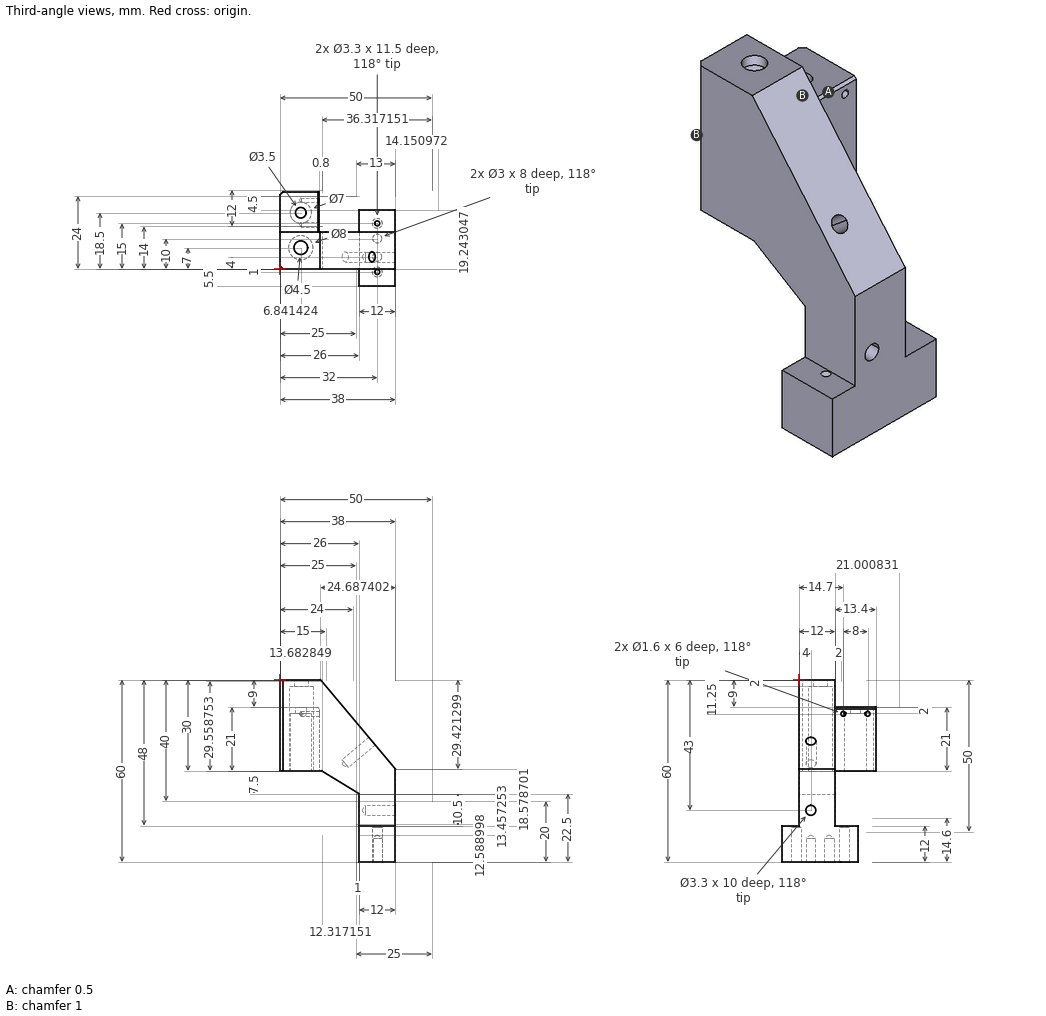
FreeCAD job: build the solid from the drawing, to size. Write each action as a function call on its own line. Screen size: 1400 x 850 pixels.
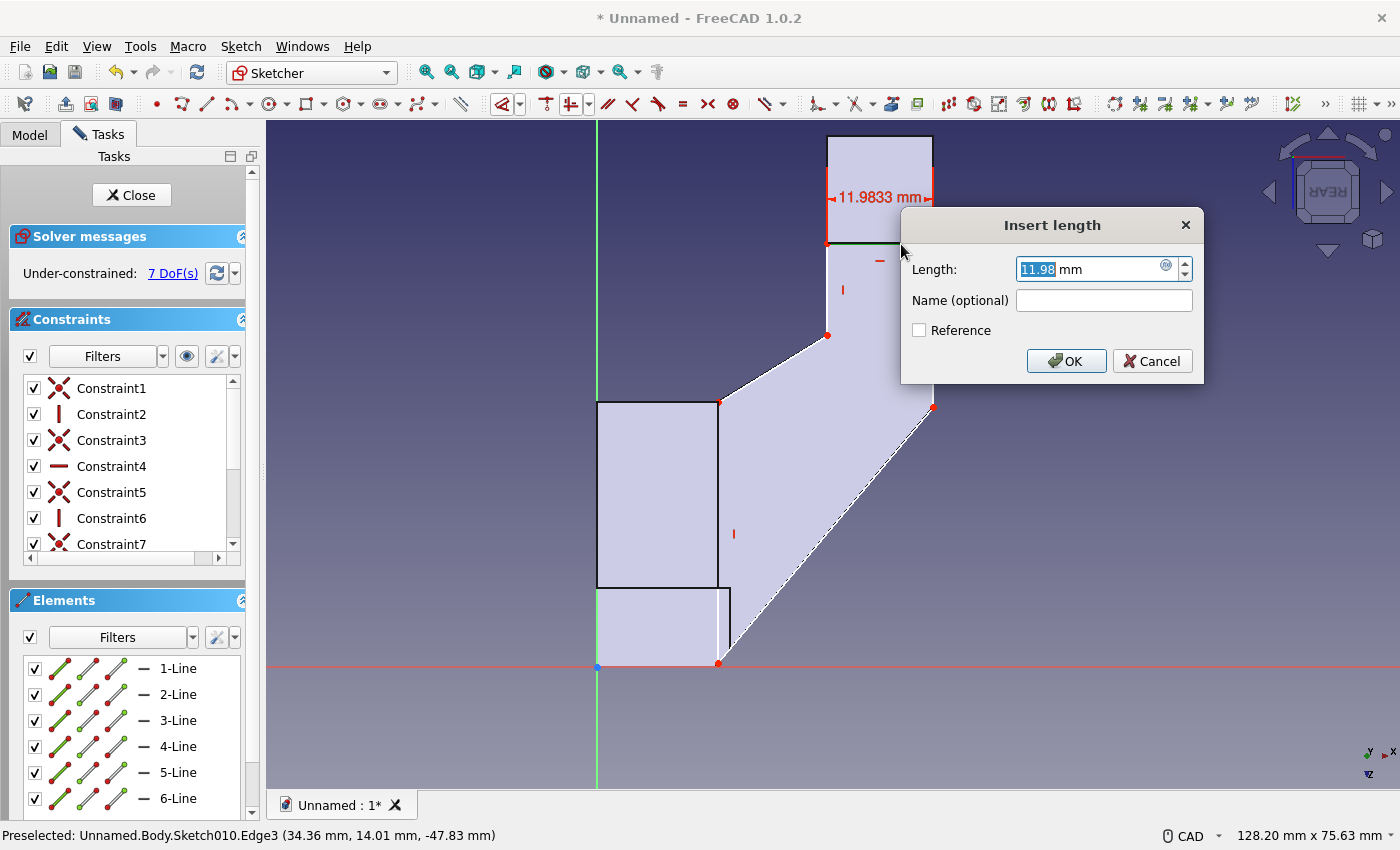
text(12)
key(Return)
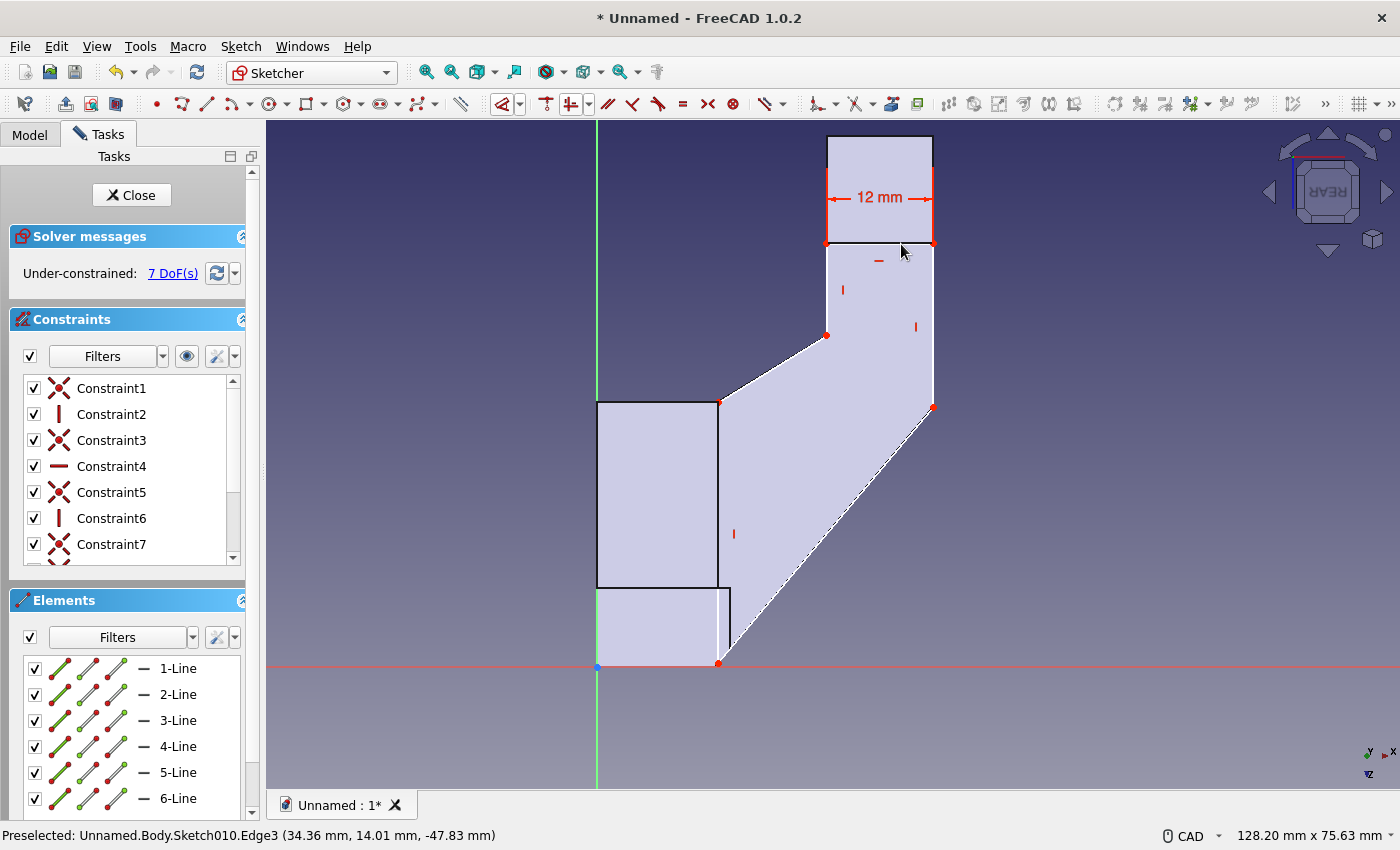
click(933, 408)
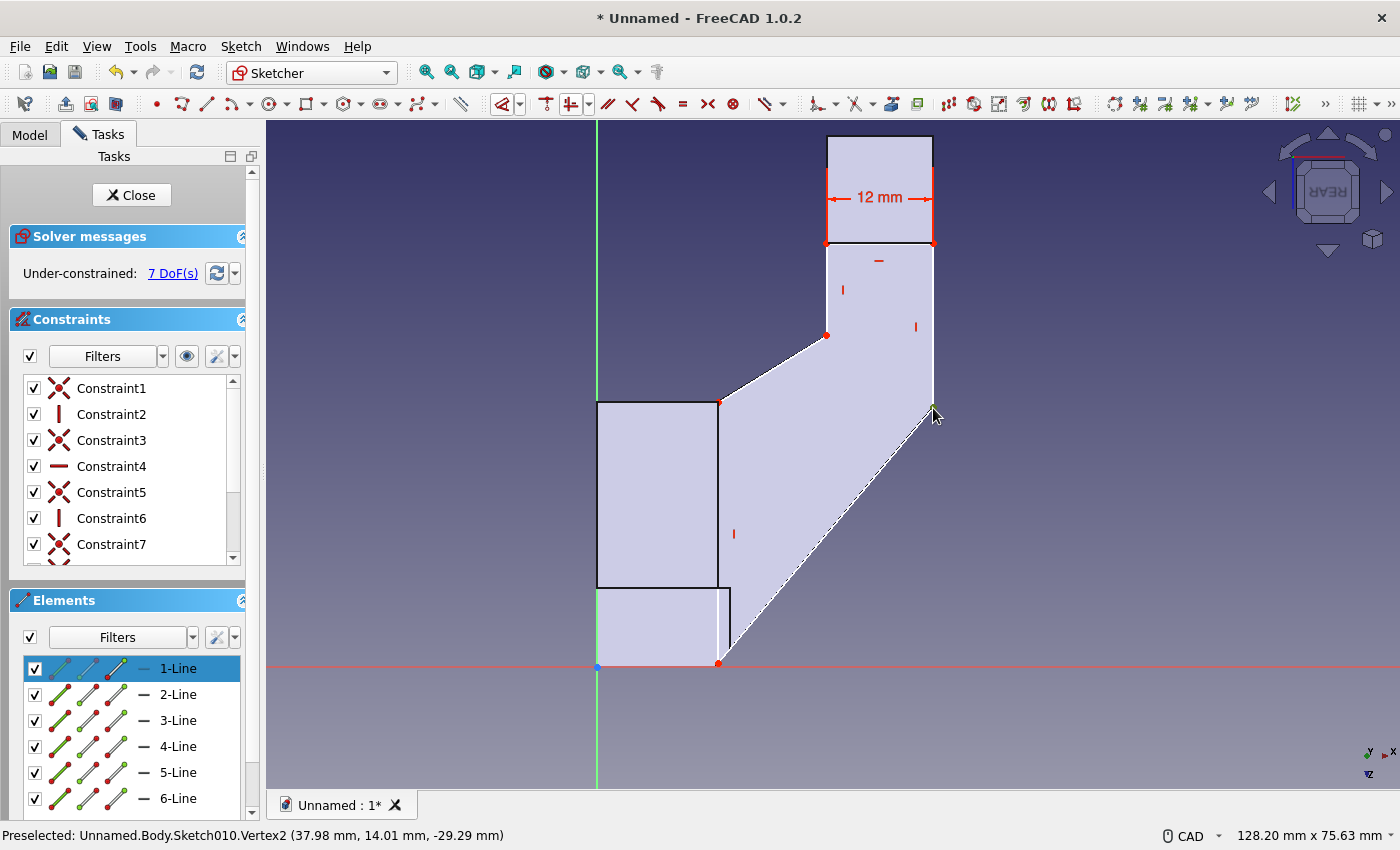
click(520, 104)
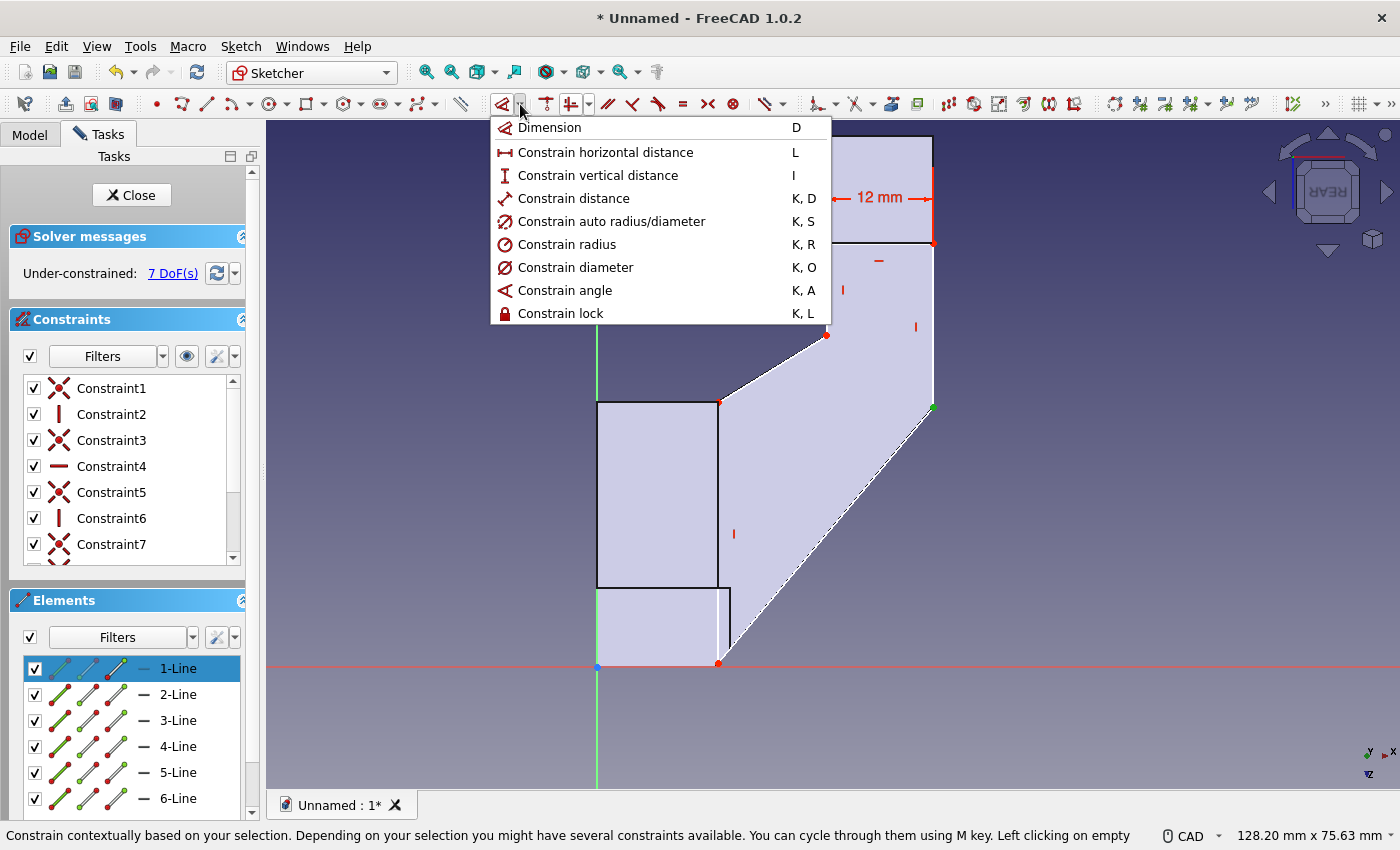
click(661, 152)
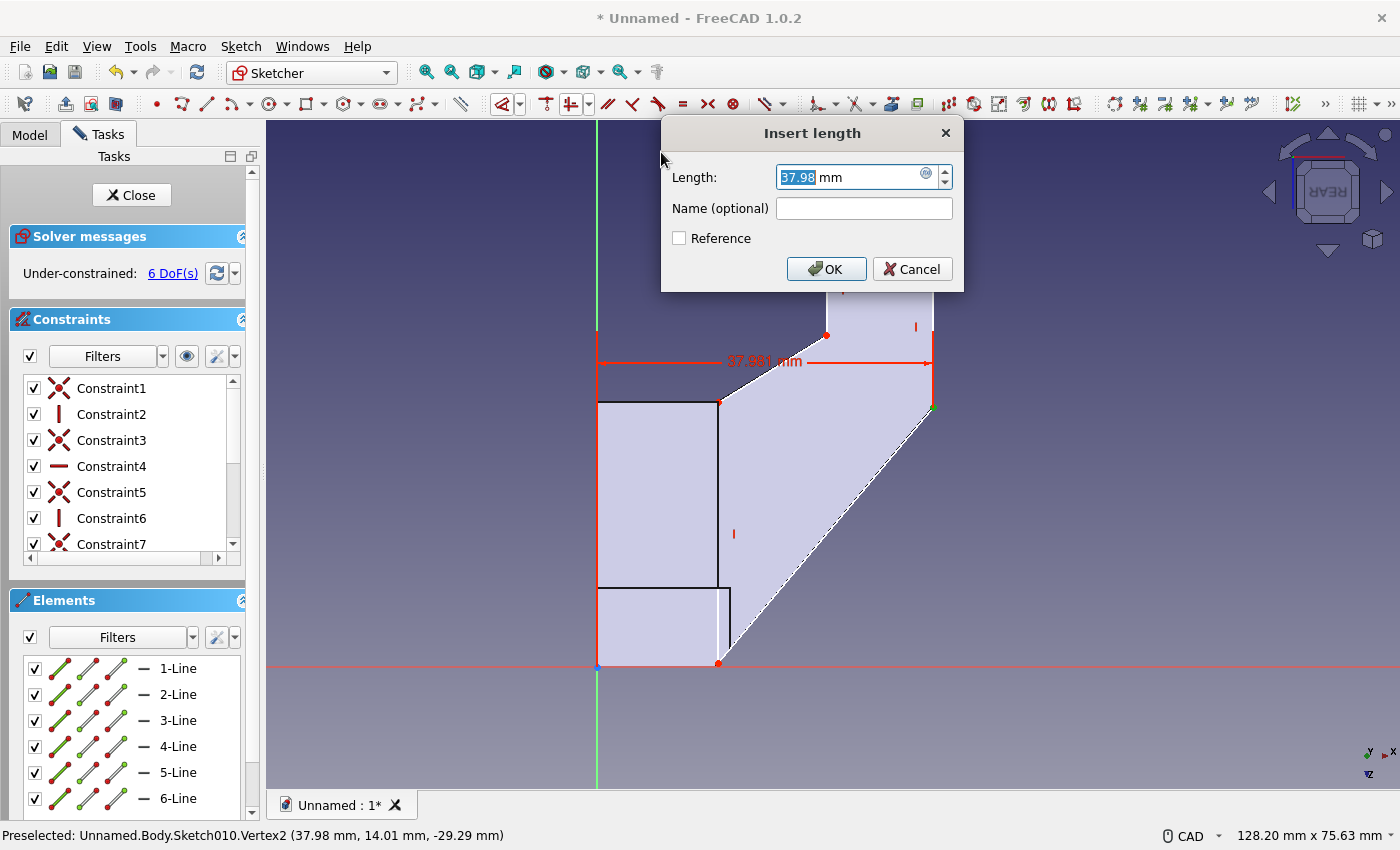
text(38)
key(Return)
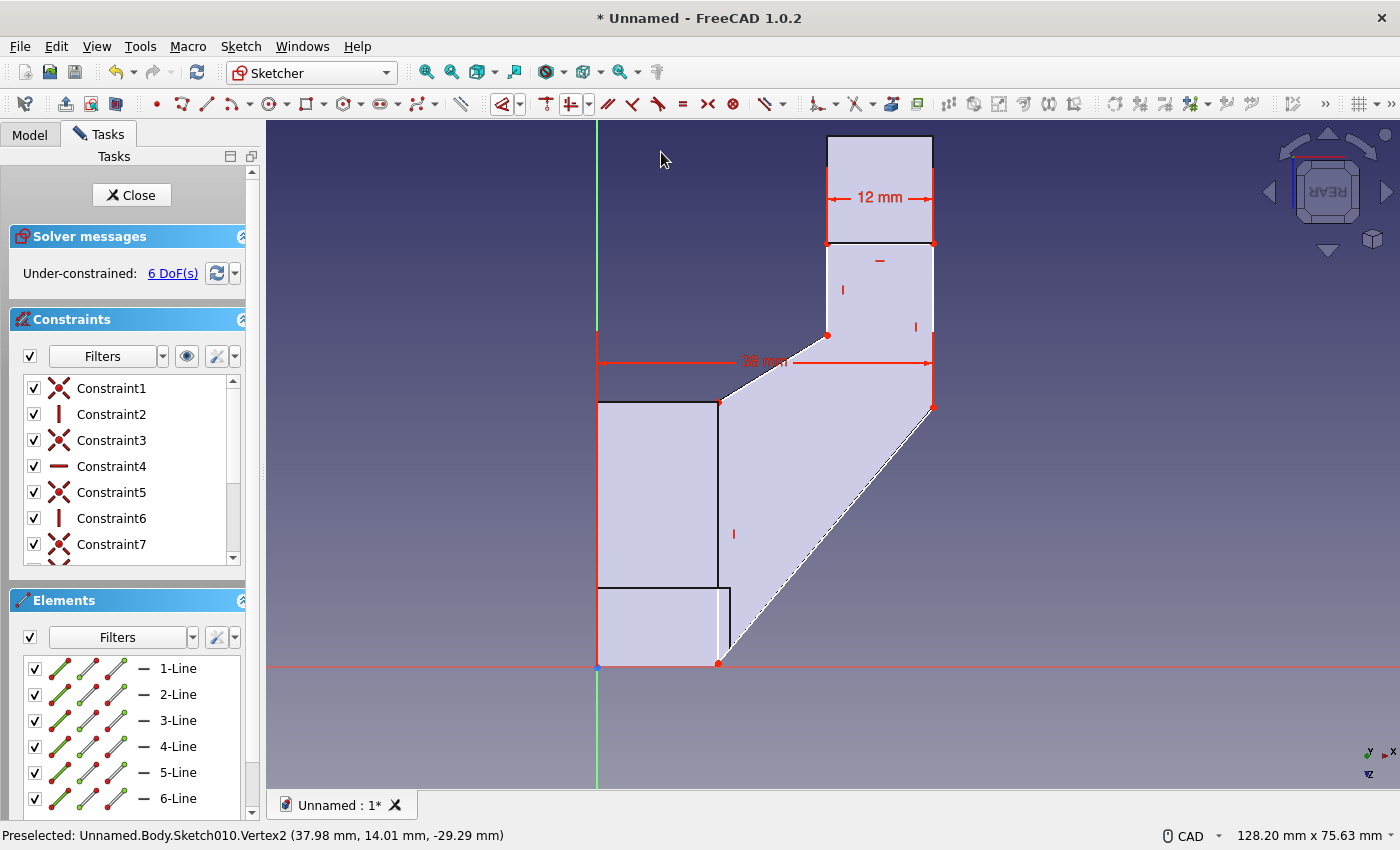
click(933, 244)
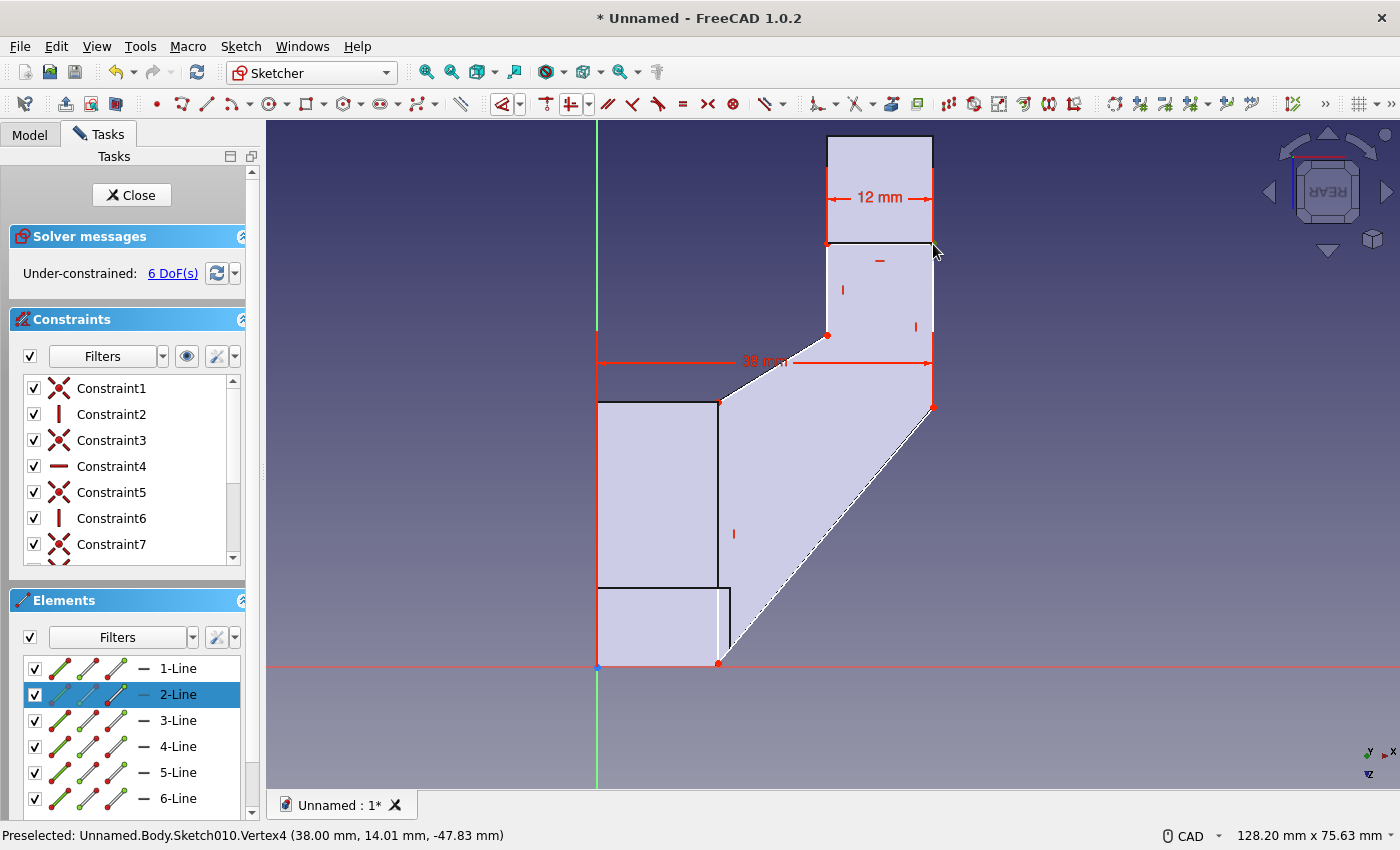
key(i)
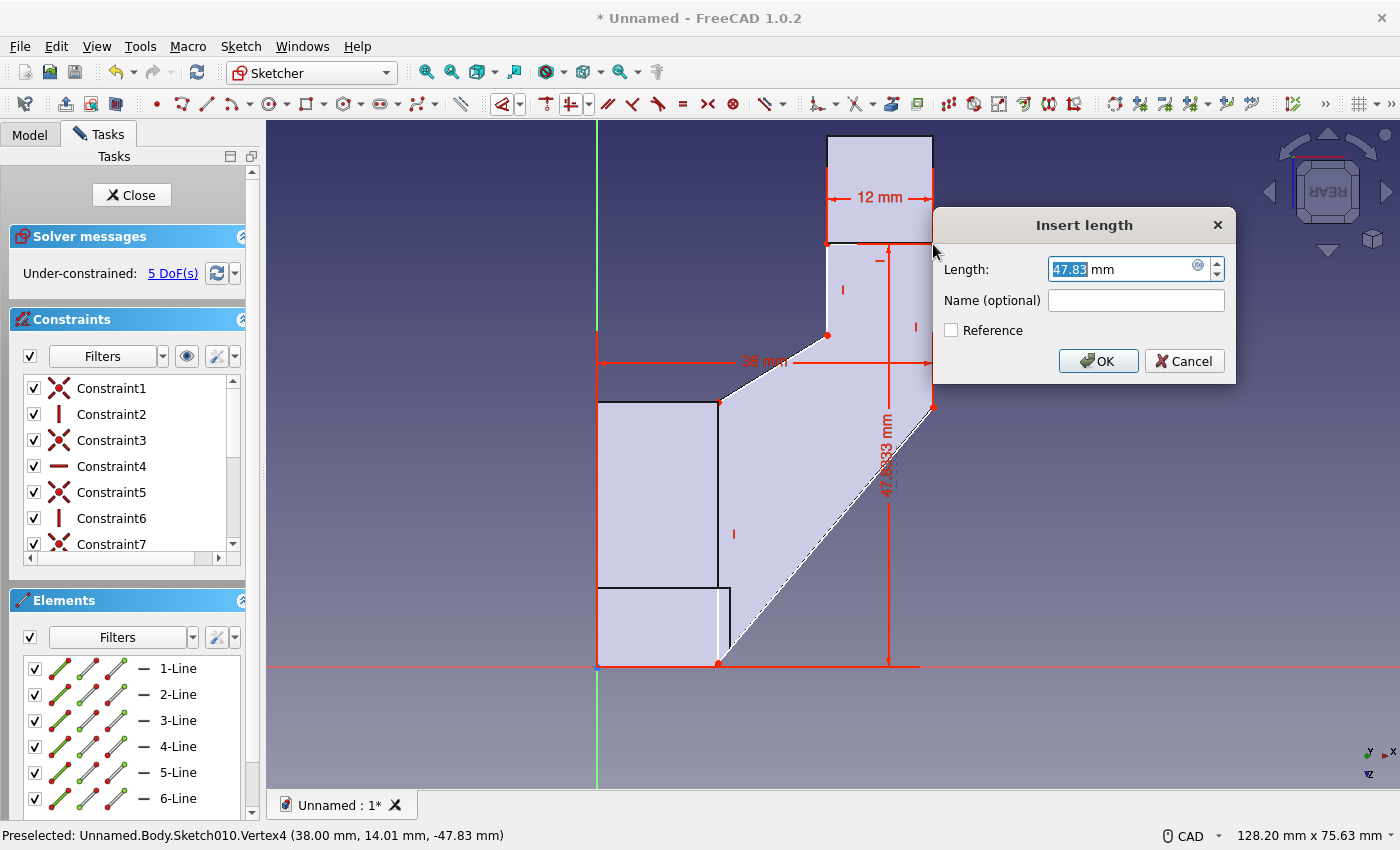
text(48)
key(Return)